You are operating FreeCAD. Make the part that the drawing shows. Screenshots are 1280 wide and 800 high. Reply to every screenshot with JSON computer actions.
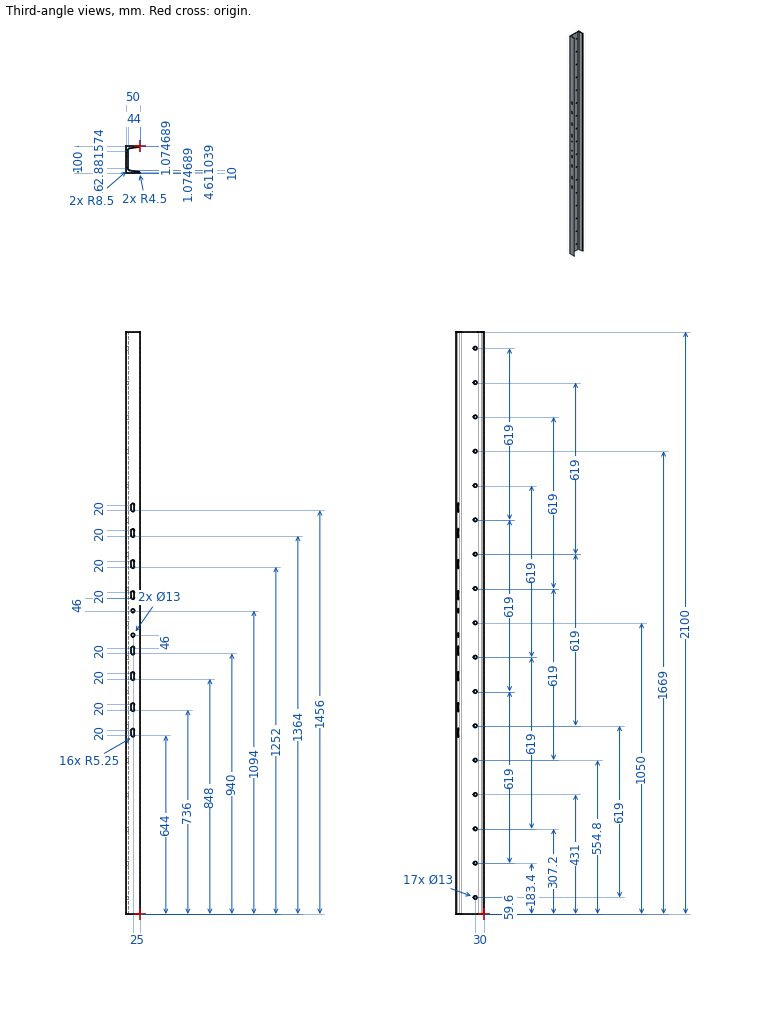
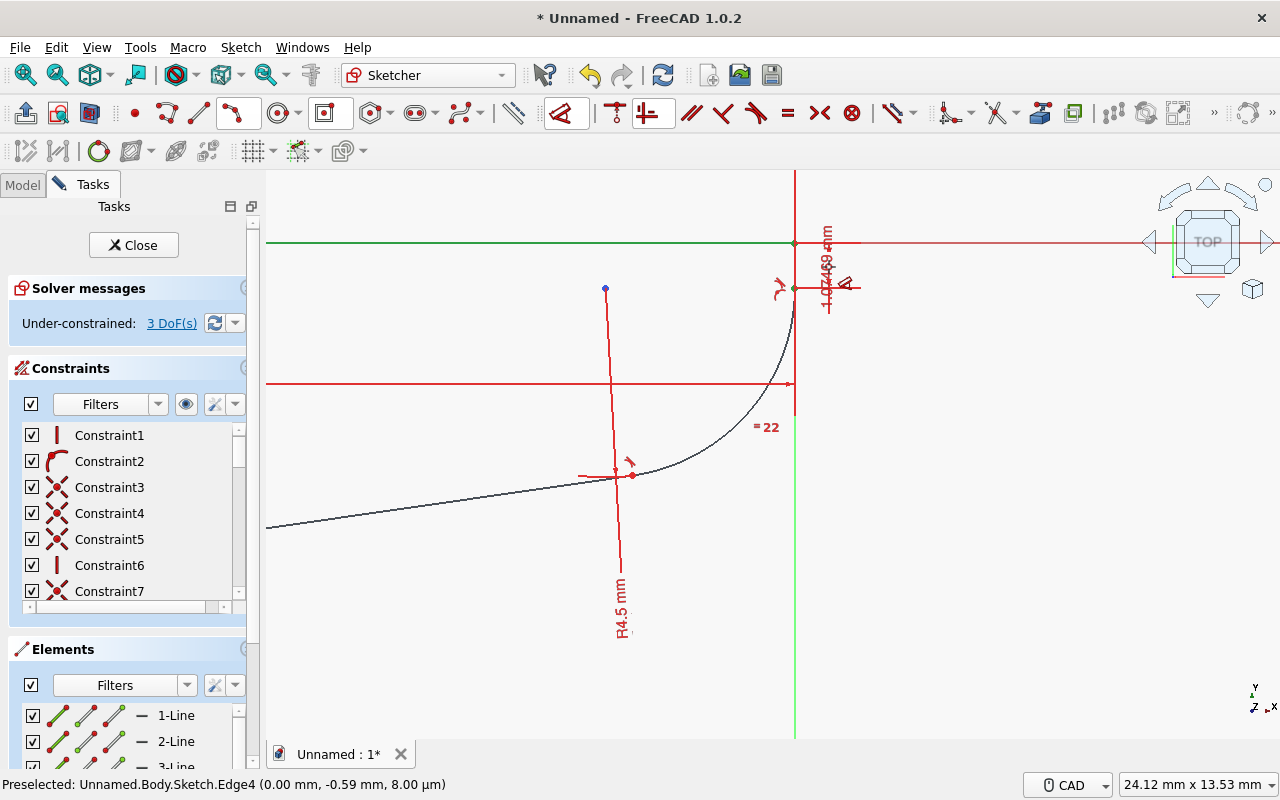
{"action": "scroll", "coordinate": [800, 266], "scroll_direction": "down", "scroll_amount": 12}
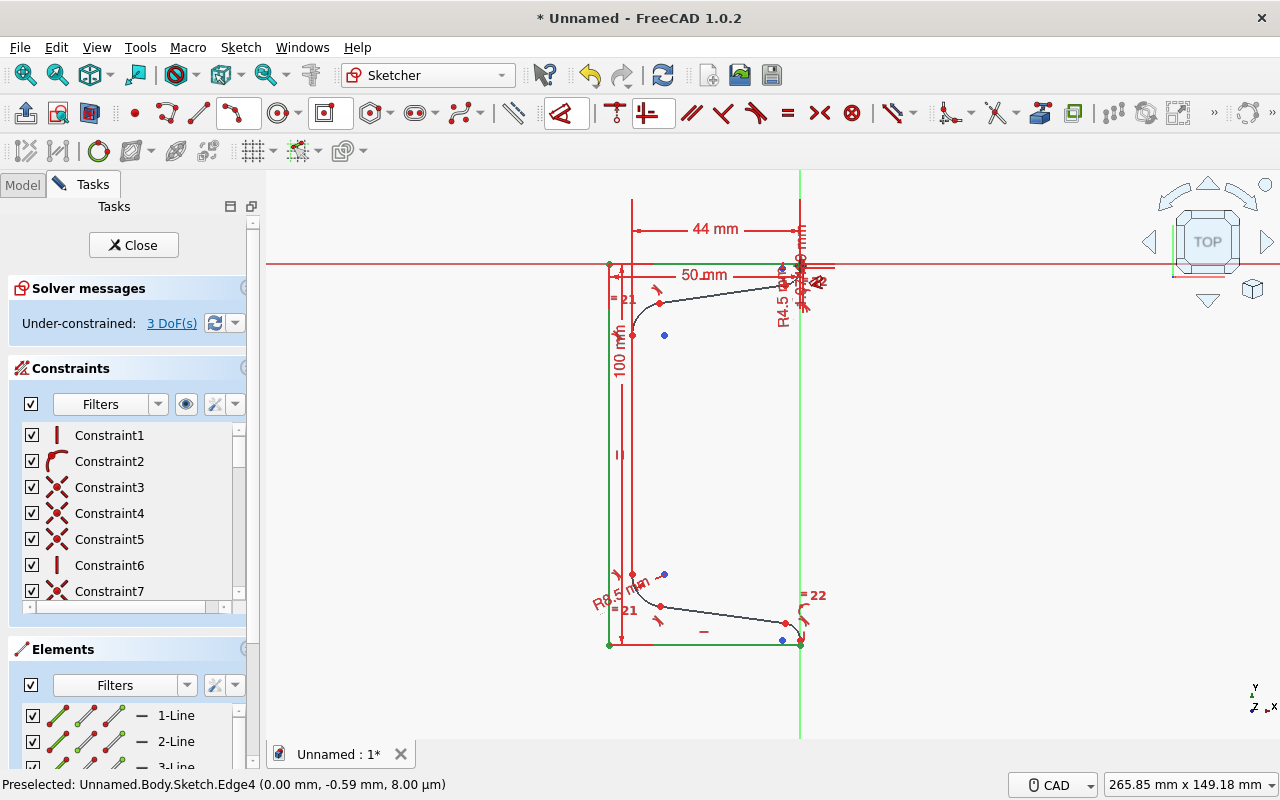
{"action": "scroll", "coordinate": [800, 644], "scroll_direction": "up", "scroll_amount": 12}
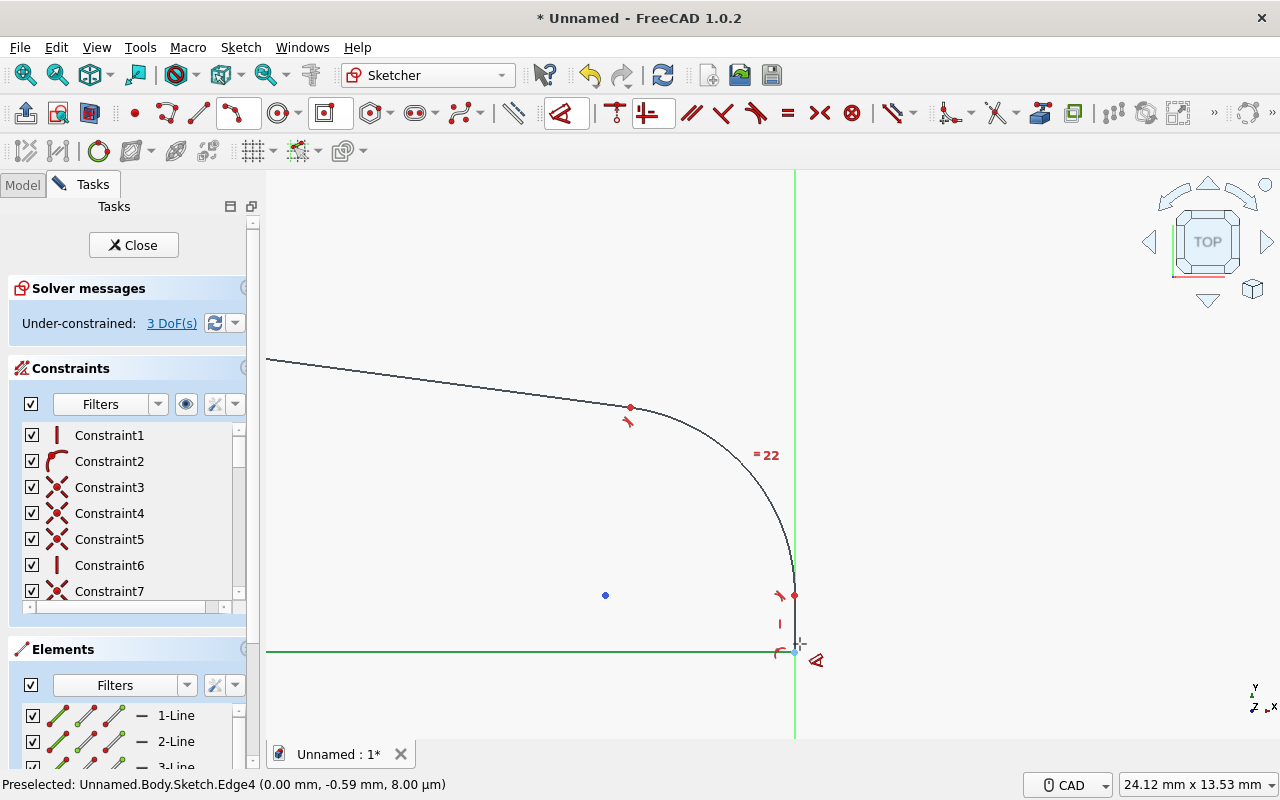
{"action": "left_click", "coordinate": [795, 635]}
{"action": "left_click", "coordinate": [829, 624]}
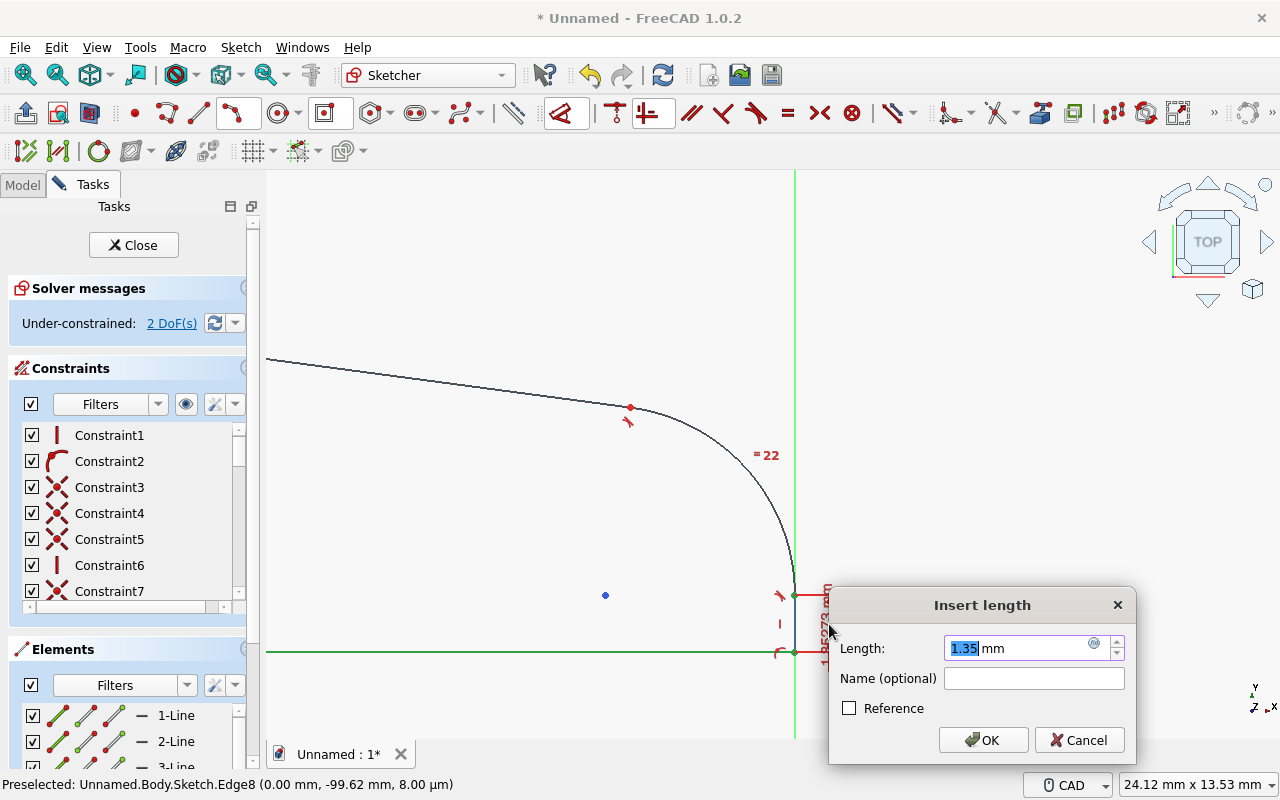
{"action": "type", "text": "1.074689"}
{"action": "key", "text": "Return"}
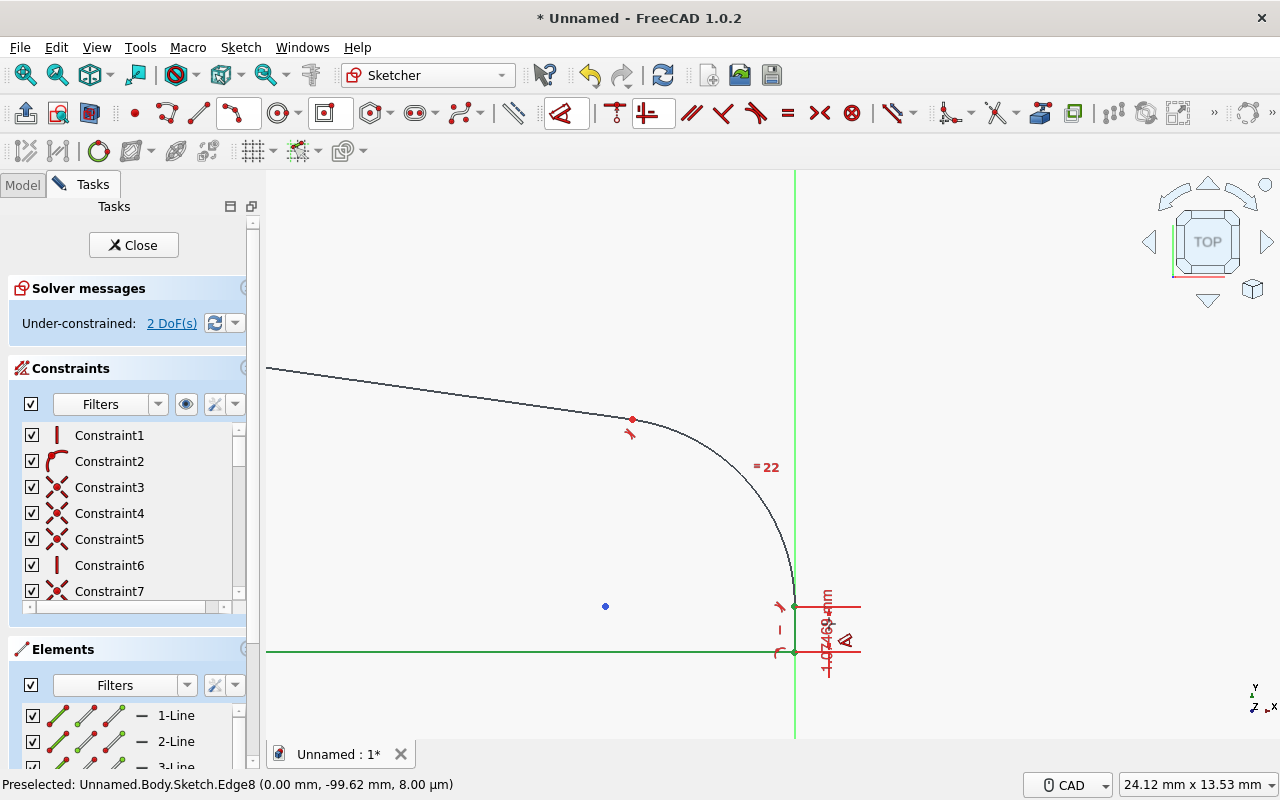
{"action": "scroll", "coordinate": [800, 645], "scroll_direction": "down", "scroll_amount": 12}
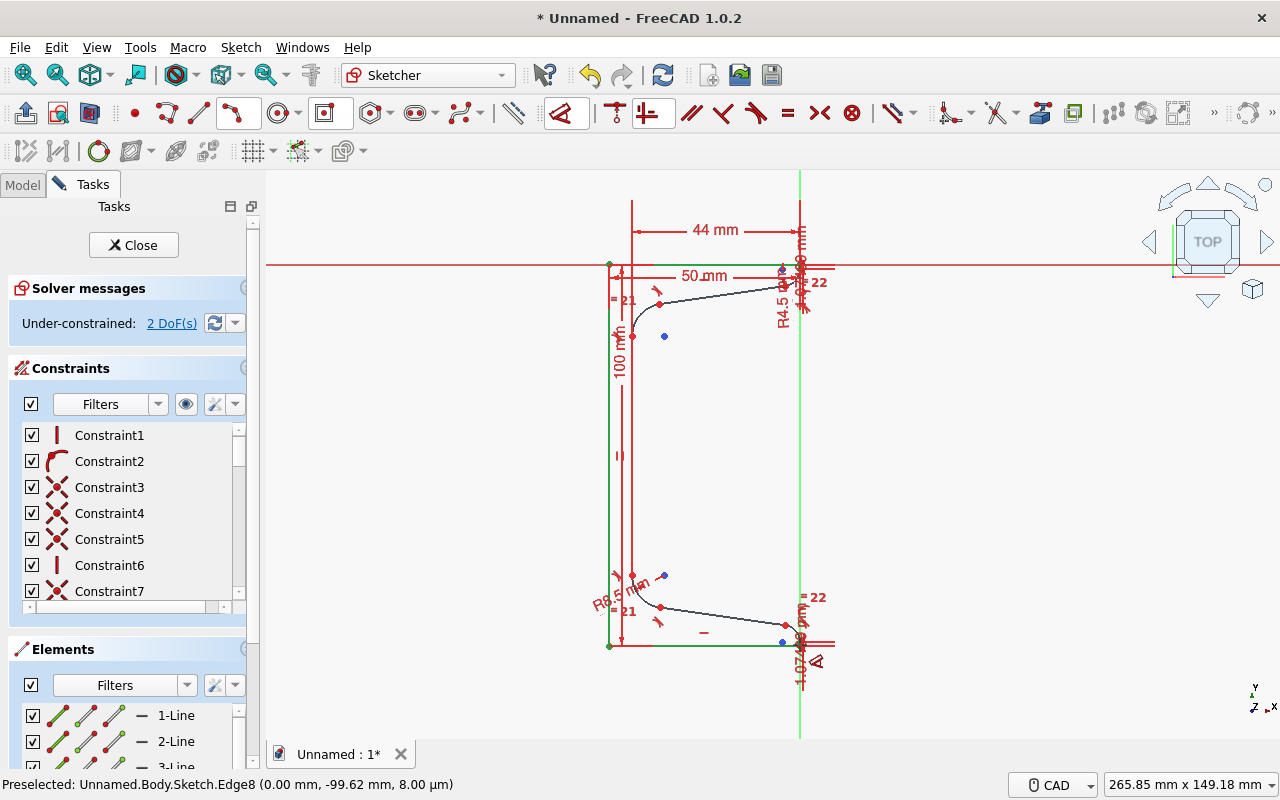
{"action": "left_click", "coordinate": [632, 504]}
{"action": "left_click", "coordinate": [666, 456]}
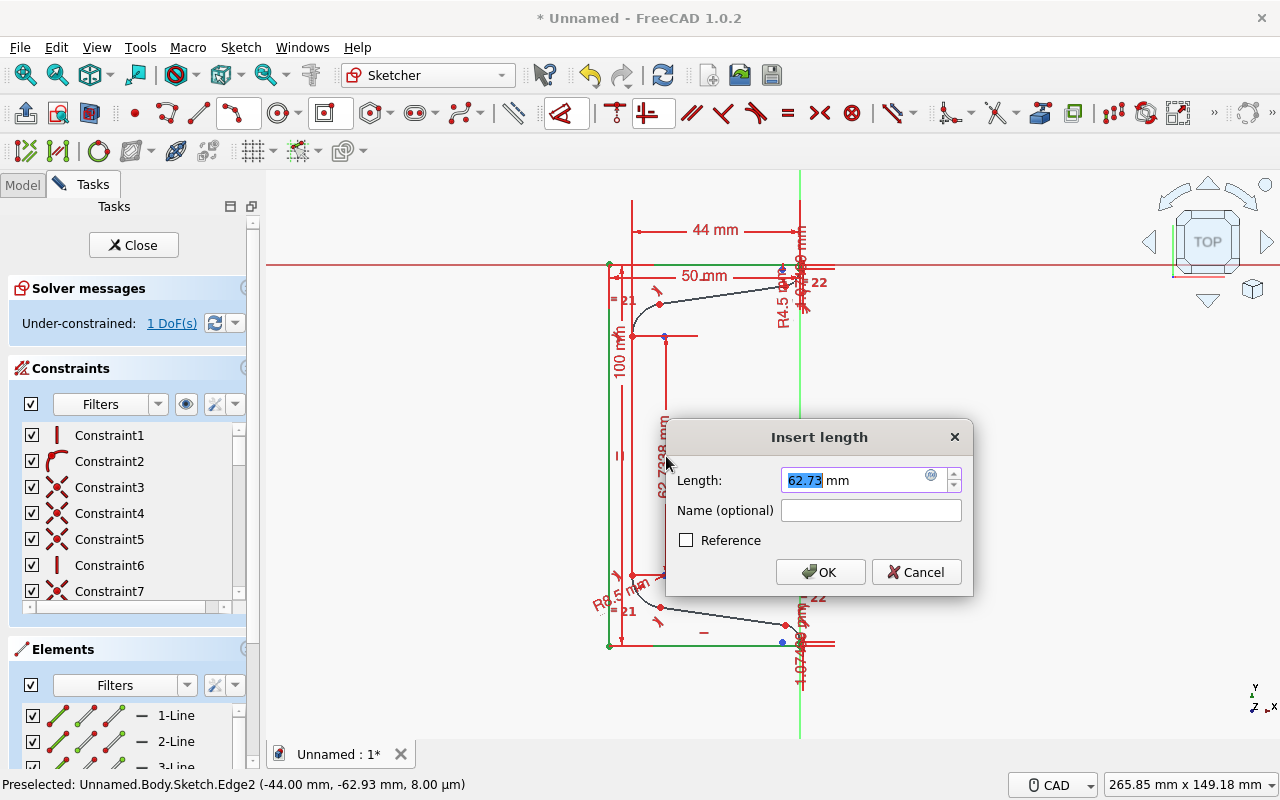
{"action": "type", "text": "62.881574"}
{"action": "key", "text": "Return"}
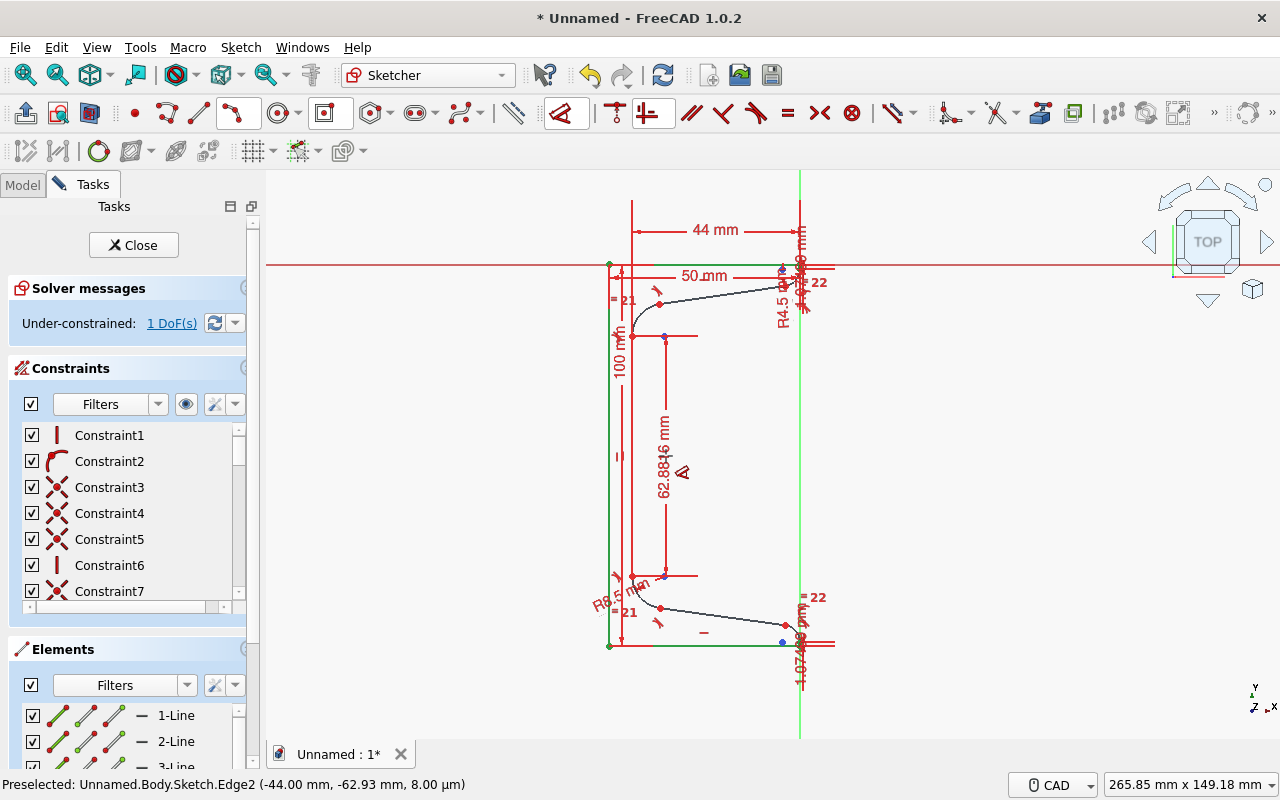
{"action": "scroll", "coordinate": [748, 620], "scroll_direction": "up", "scroll_amount": 5}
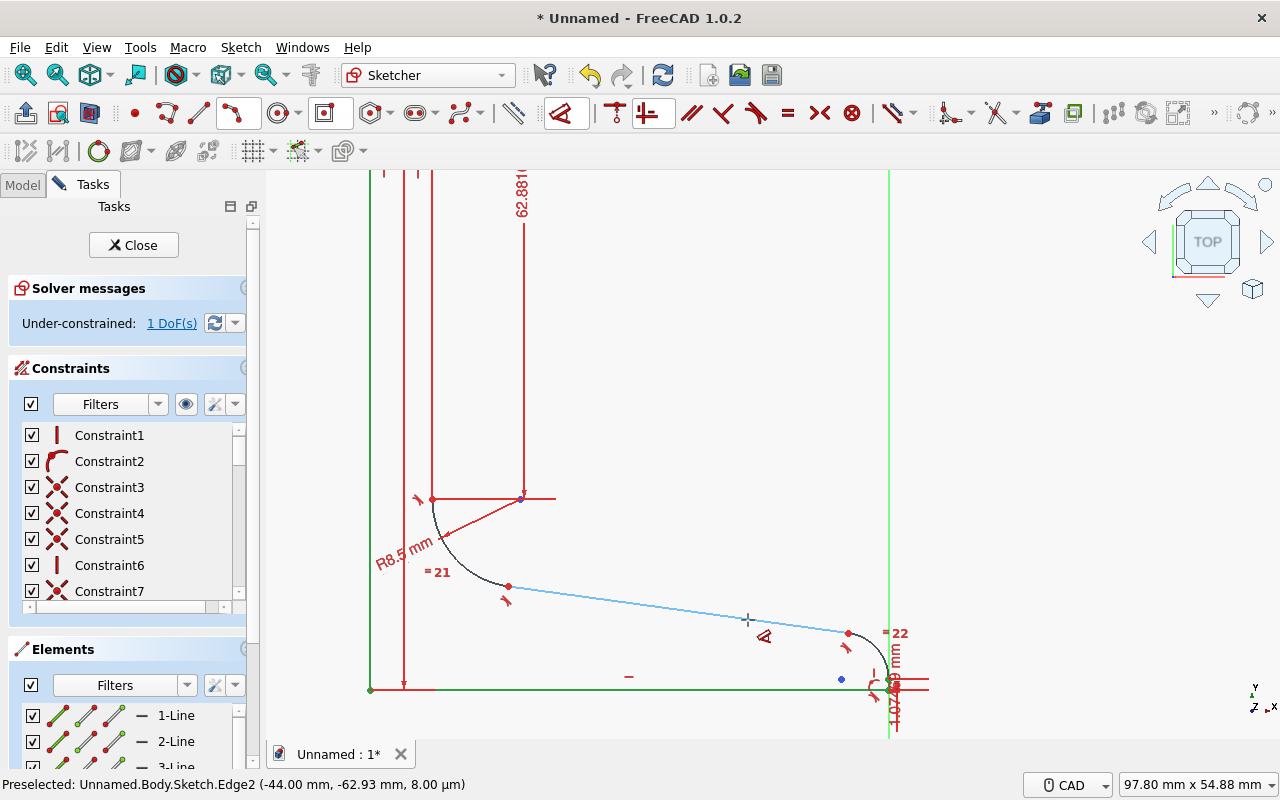
{"action": "left_click", "coordinate": [746, 619]}
{"action": "left_click", "coordinate": [475, 610]}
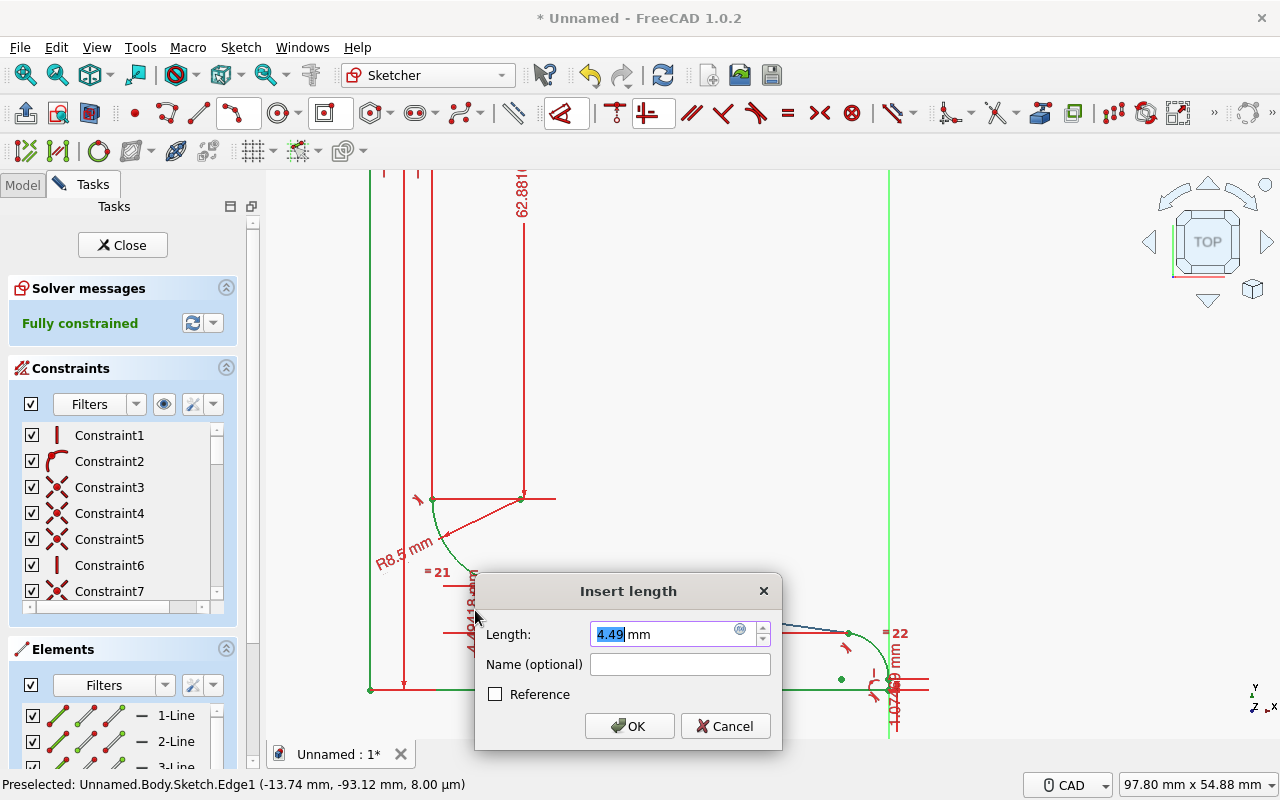
{"action": "type", "text": "4.611039"}
{"action": "key", "text": "Return"}
{"action": "key", "text": "Escape"}